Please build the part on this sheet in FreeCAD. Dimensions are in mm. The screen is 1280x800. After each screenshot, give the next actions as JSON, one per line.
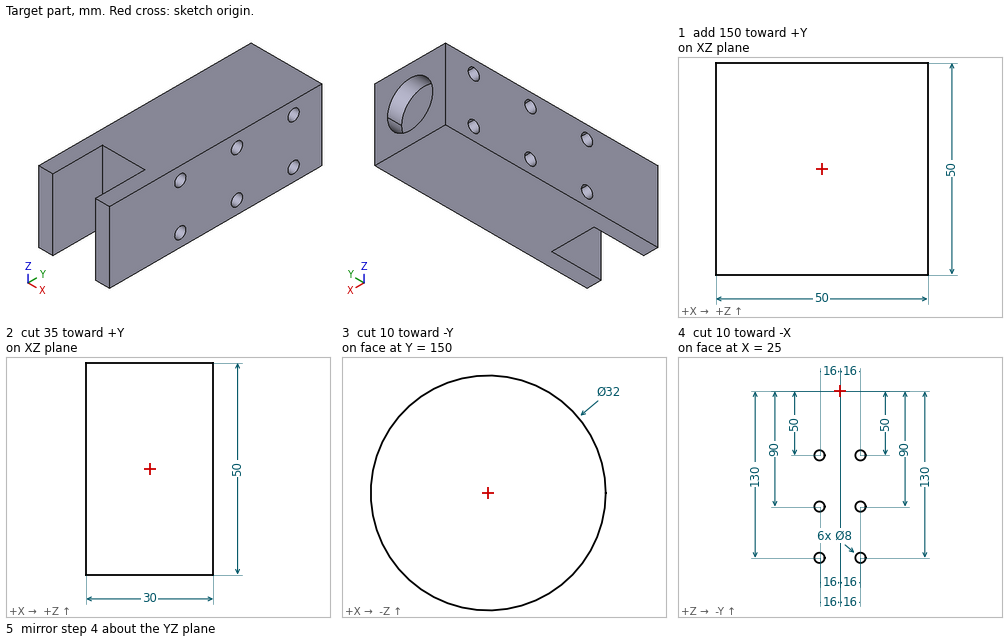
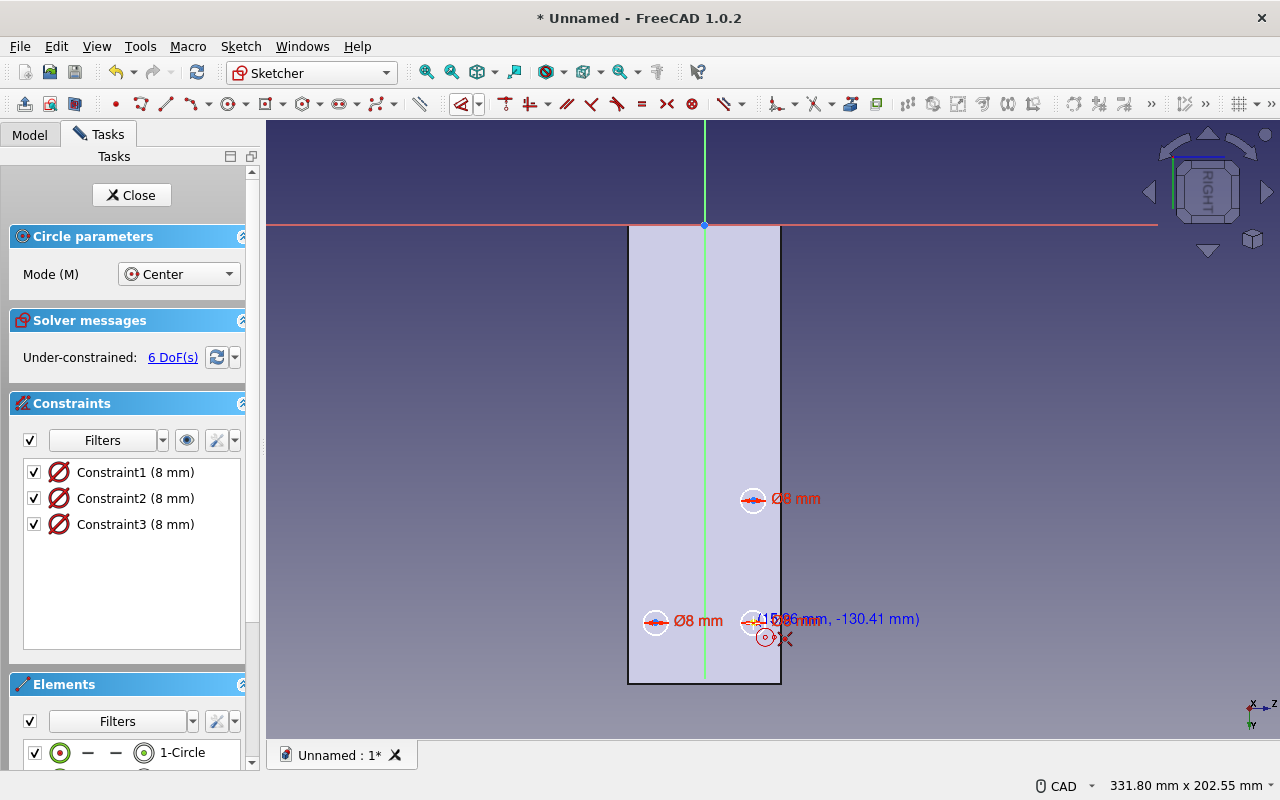
{"action": "scroll", "coordinate": [753, 378], "scroll_direction": "up", "scroll_amount": 4}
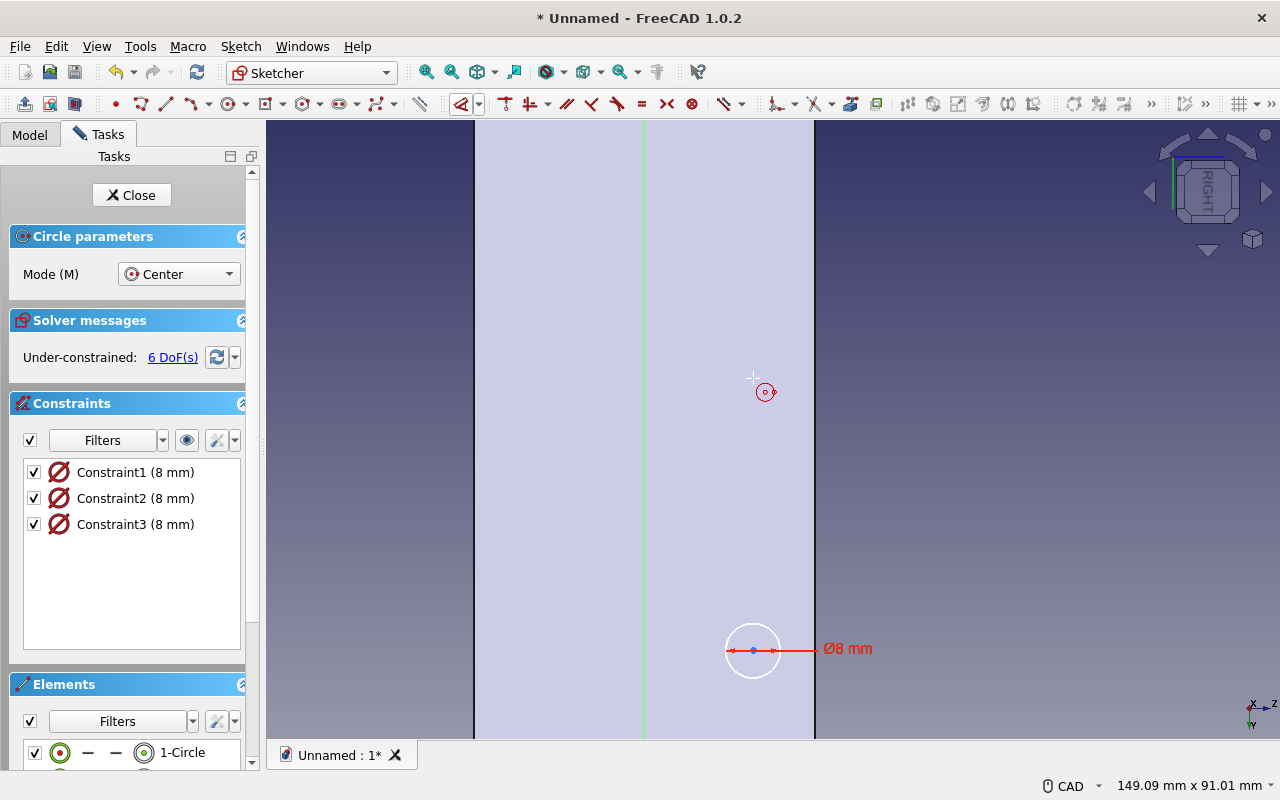
{"action": "left_click", "coordinate": [753, 378]}
{"action": "mouse_move", "coordinate": [773, 359]}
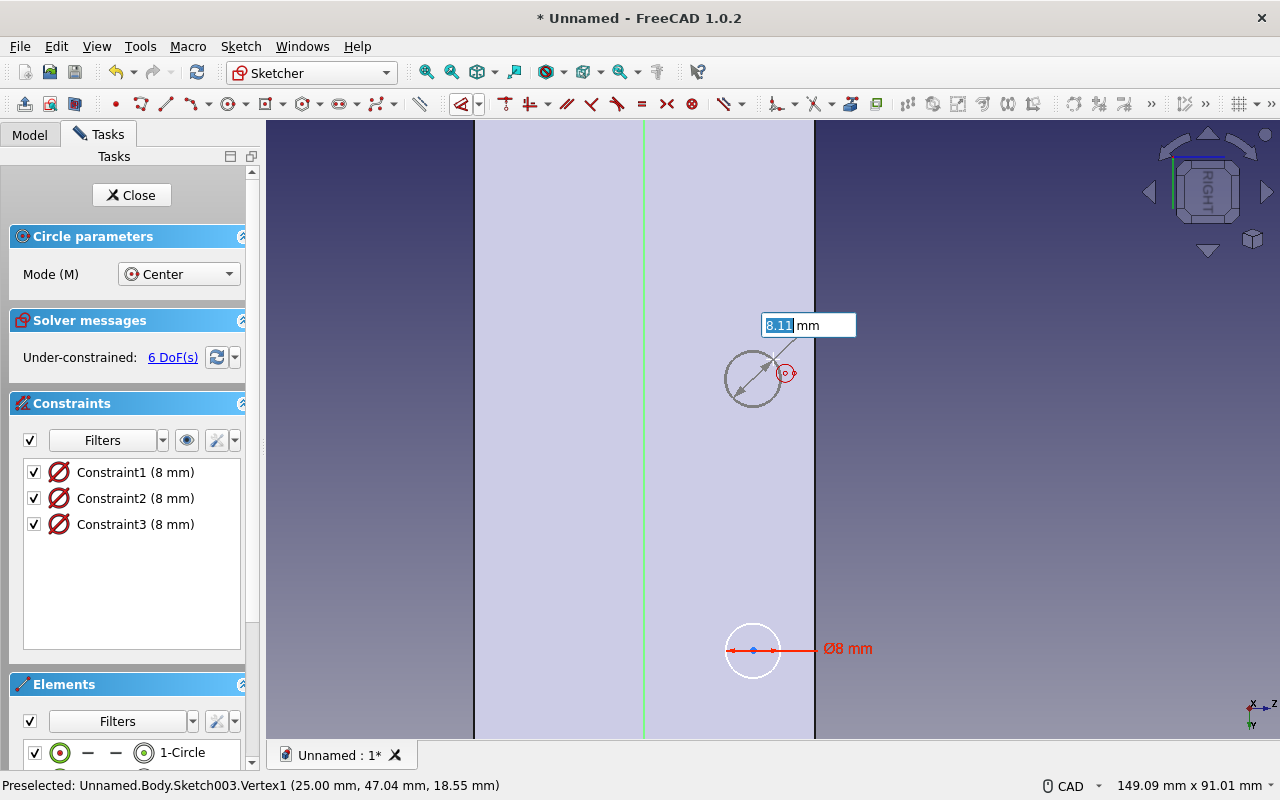
{"action": "type", "text": "8"}
{"action": "key", "text": "Return"}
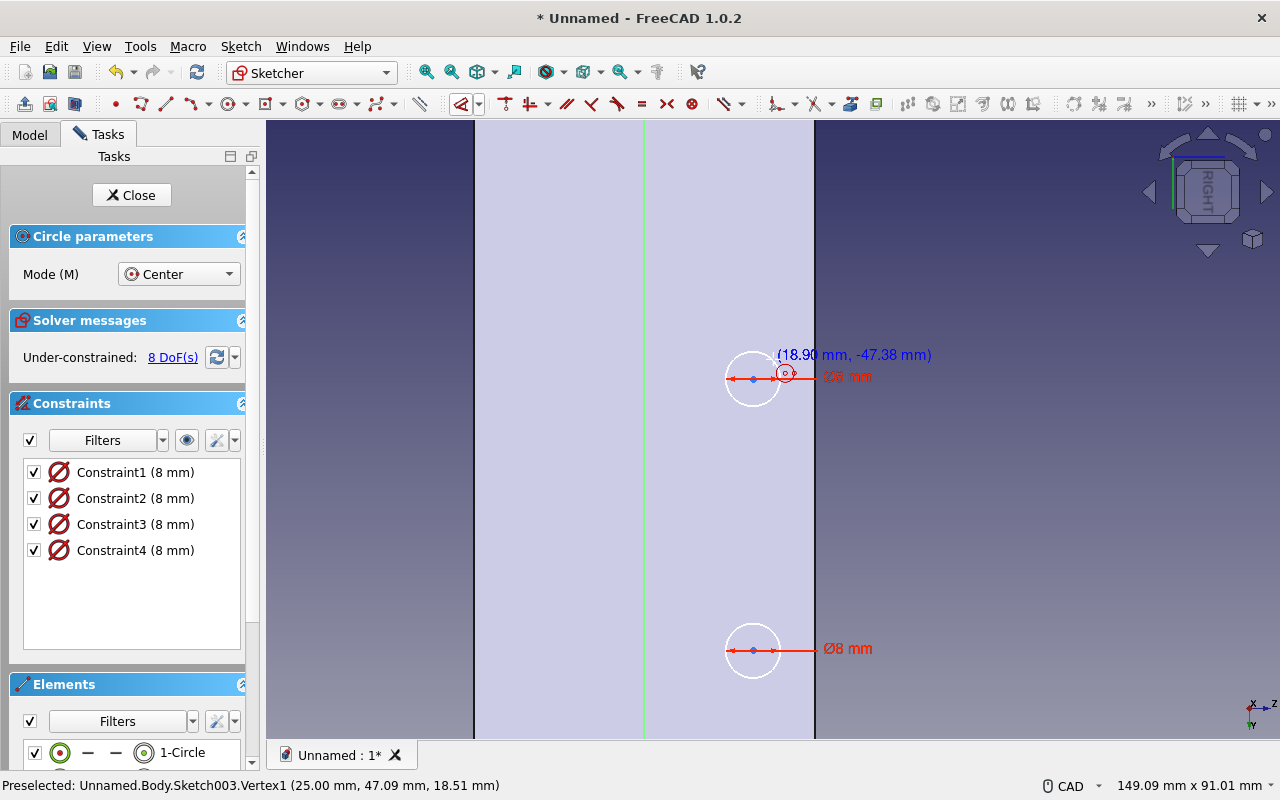
{"action": "left_click", "coordinate": [536, 378]}
{"action": "mouse_move", "coordinate": [555, 359]}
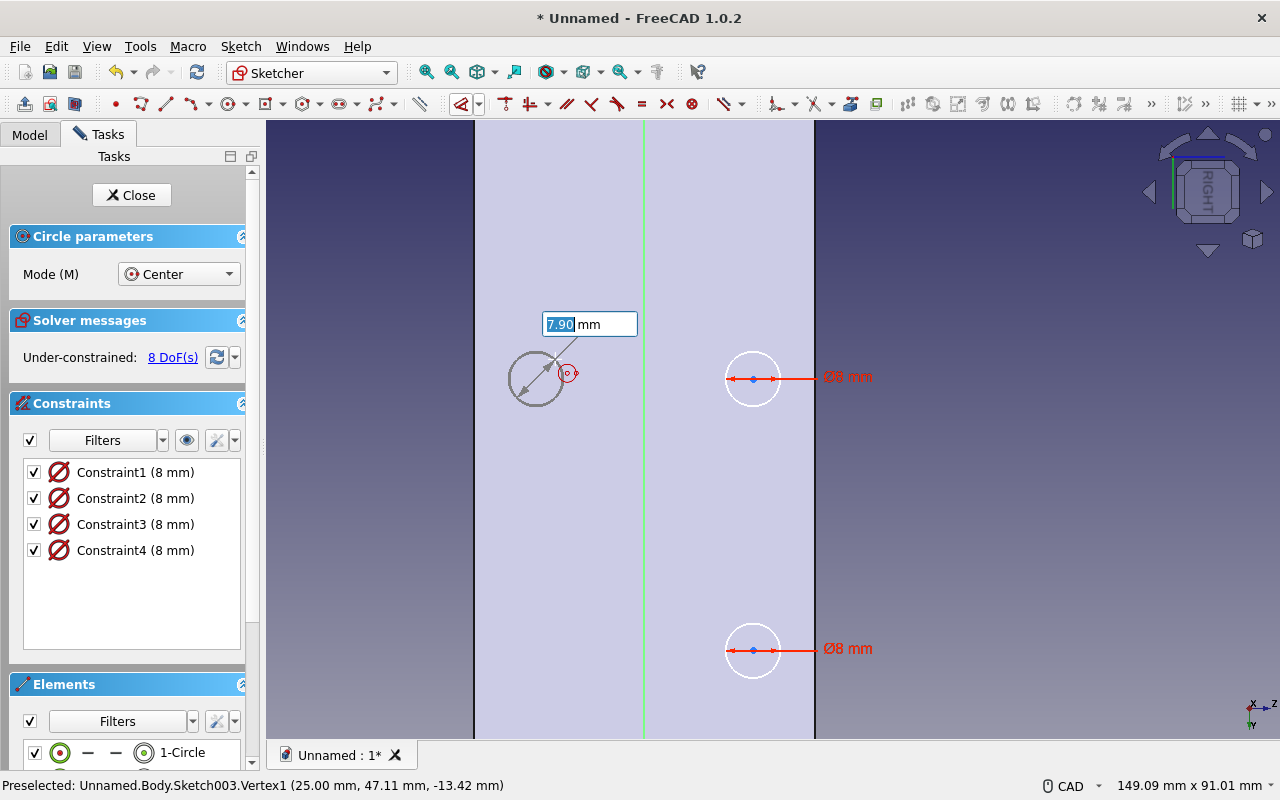
{"action": "type", "text": "8"}
{"action": "key", "text": "Return"}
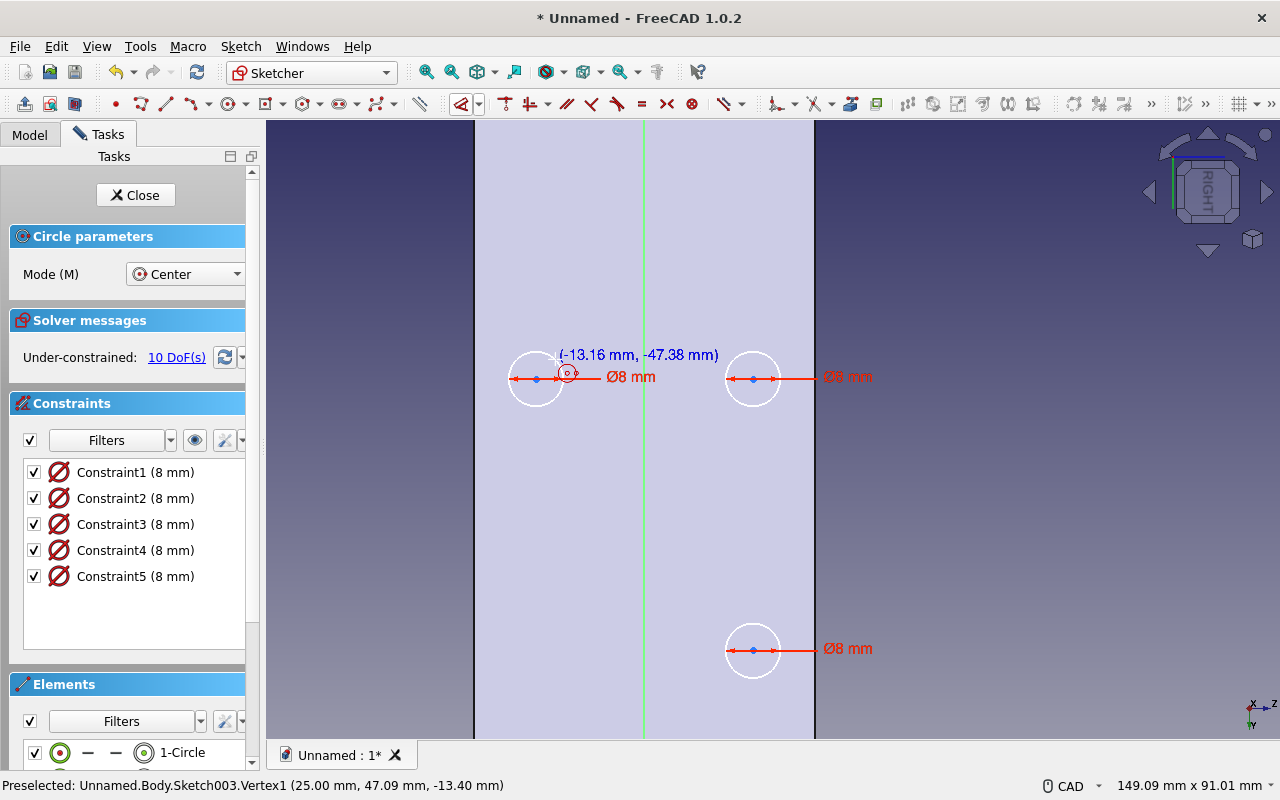
{"action": "left_click", "coordinate": [536, 650]}
{"action": "mouse_move", "coordinate": [555, 631]}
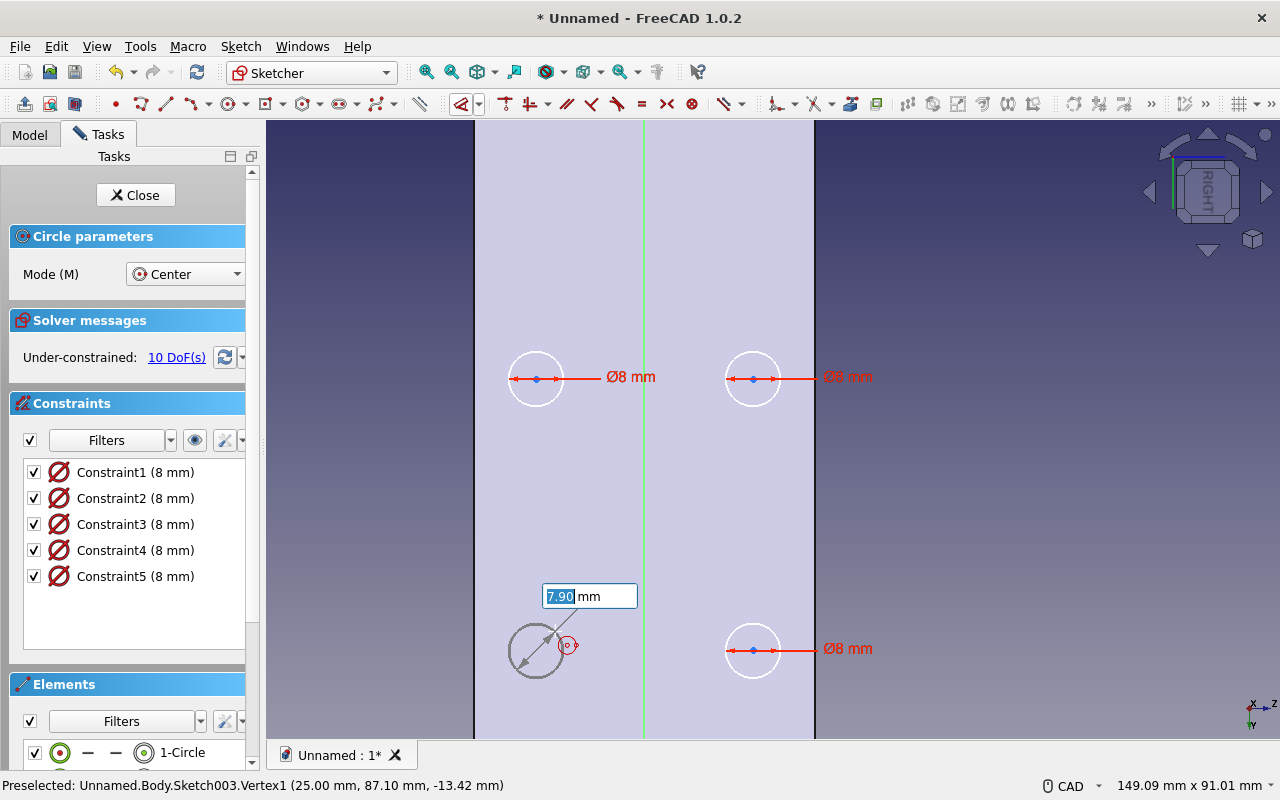
{"action": "type", "text": "8"}
{"action": "key", "text": "Return"}
{"action": "key", "text": "Escape"}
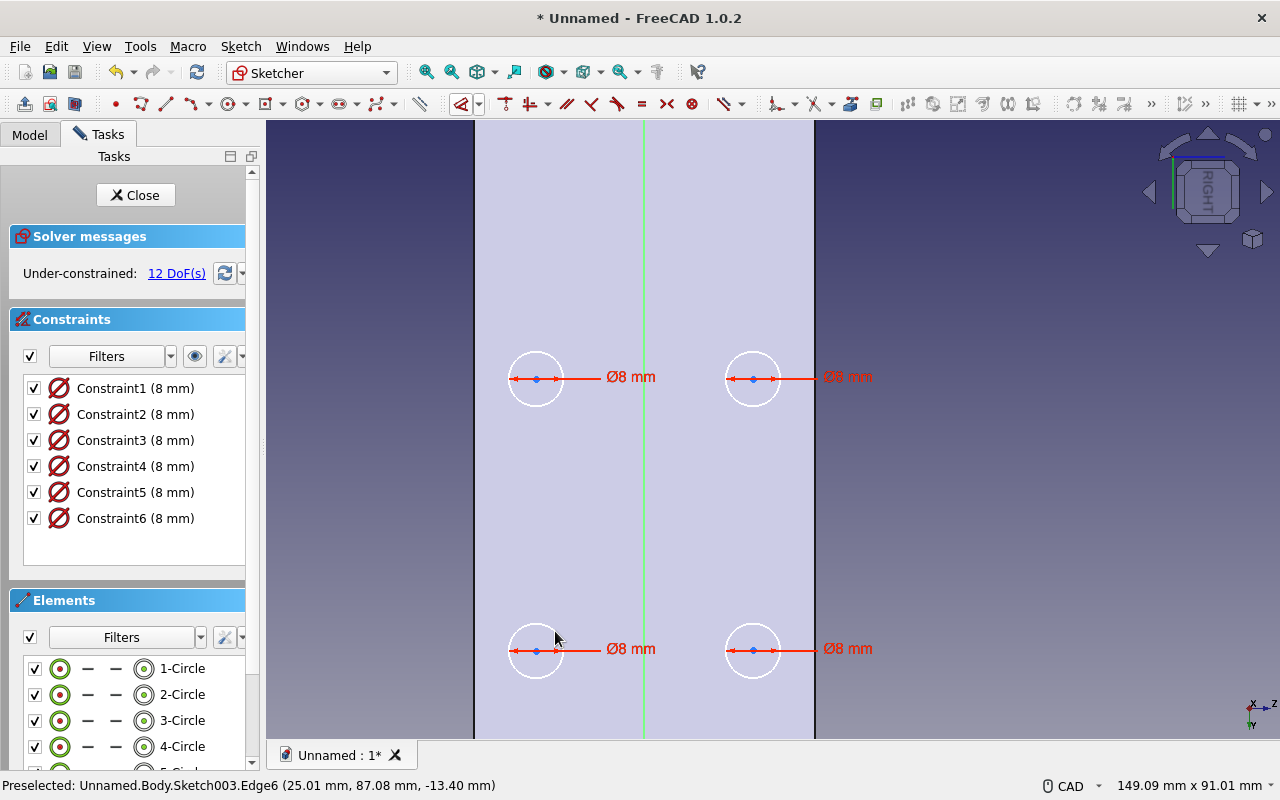
{"action": "left_click", "coordinate": [460, 104]}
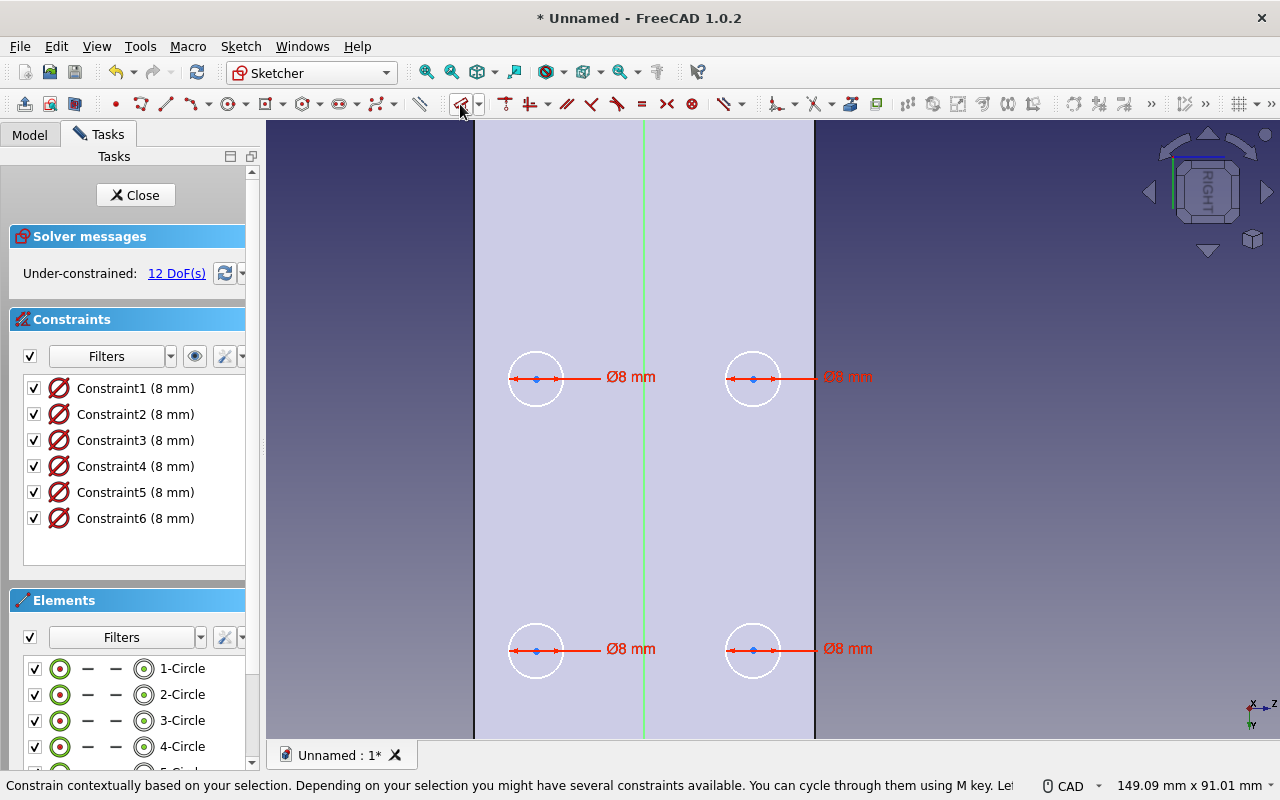
{"action": "scroll", "coordinate": [753, 377], "scroll_direction": "down", "scroll_amount": 4}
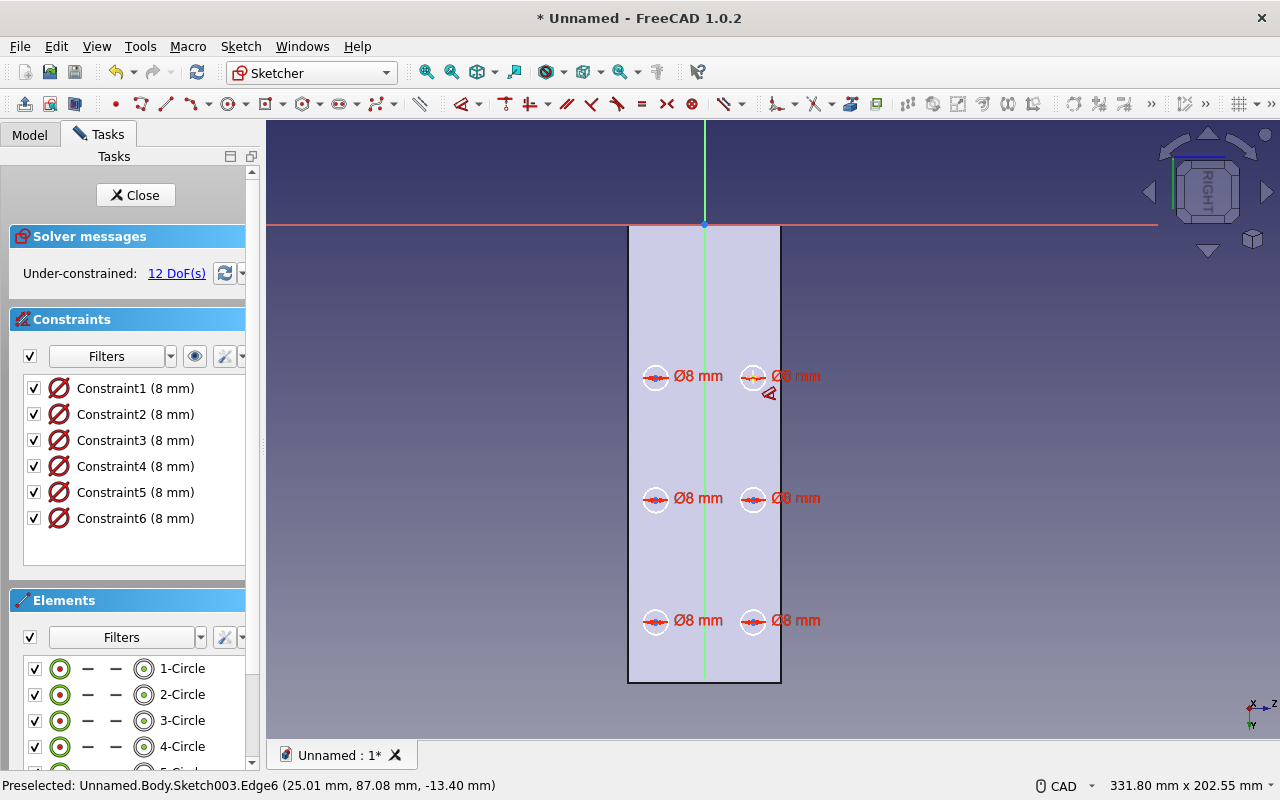
{"action": "left_click", "coordinate": [753, 622]}
{"action": "left_click", "coordinate": [729, 191]}